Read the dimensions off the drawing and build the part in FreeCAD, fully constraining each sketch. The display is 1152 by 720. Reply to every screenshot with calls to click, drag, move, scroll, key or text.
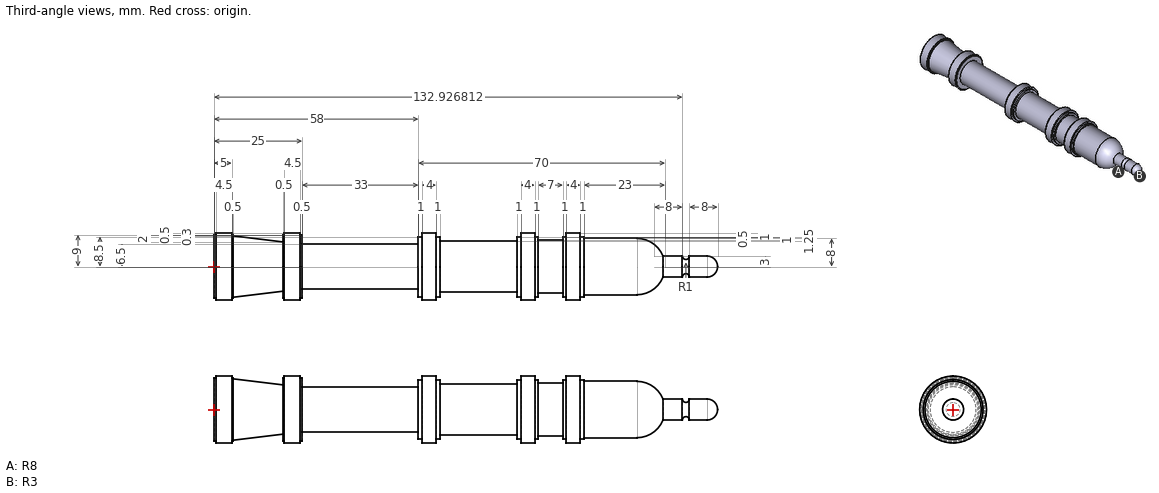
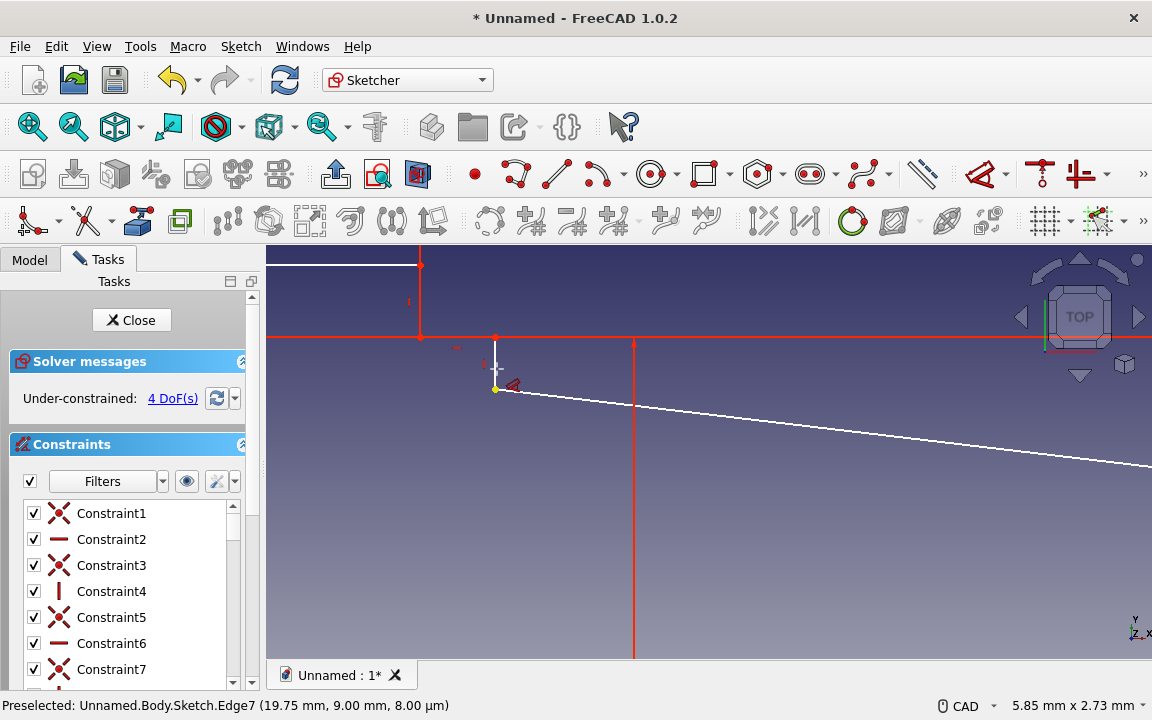
click(495, 369)
click(461, 363)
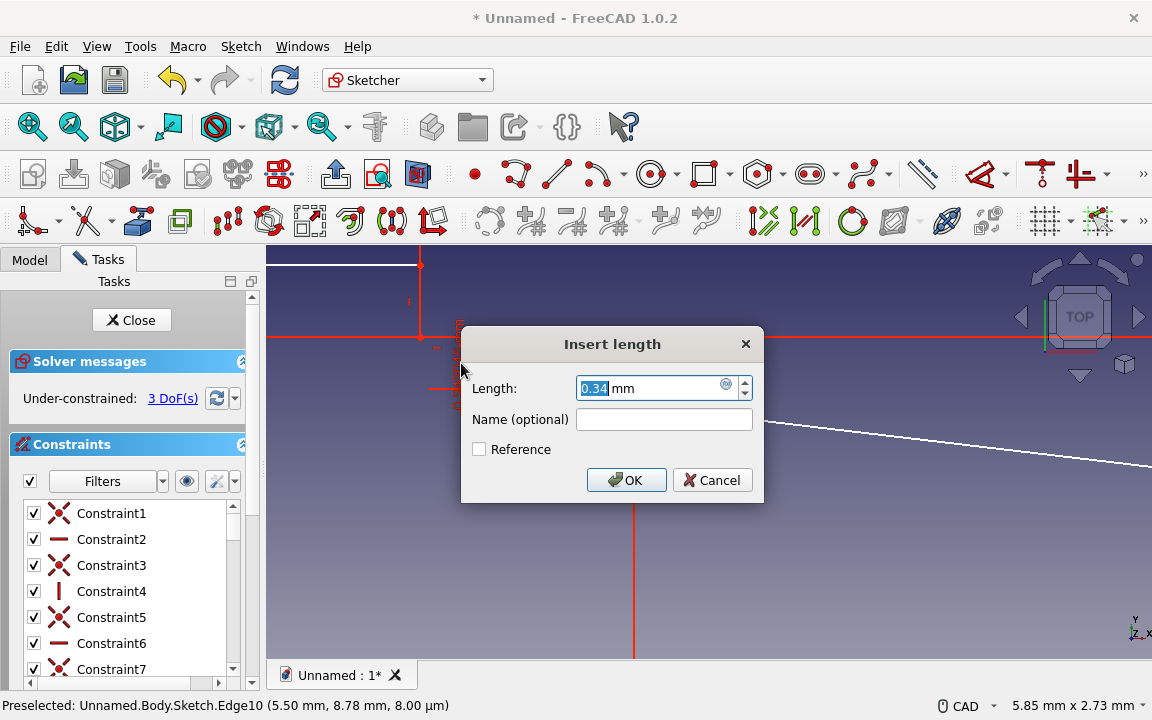
text(0.3)
key(Return)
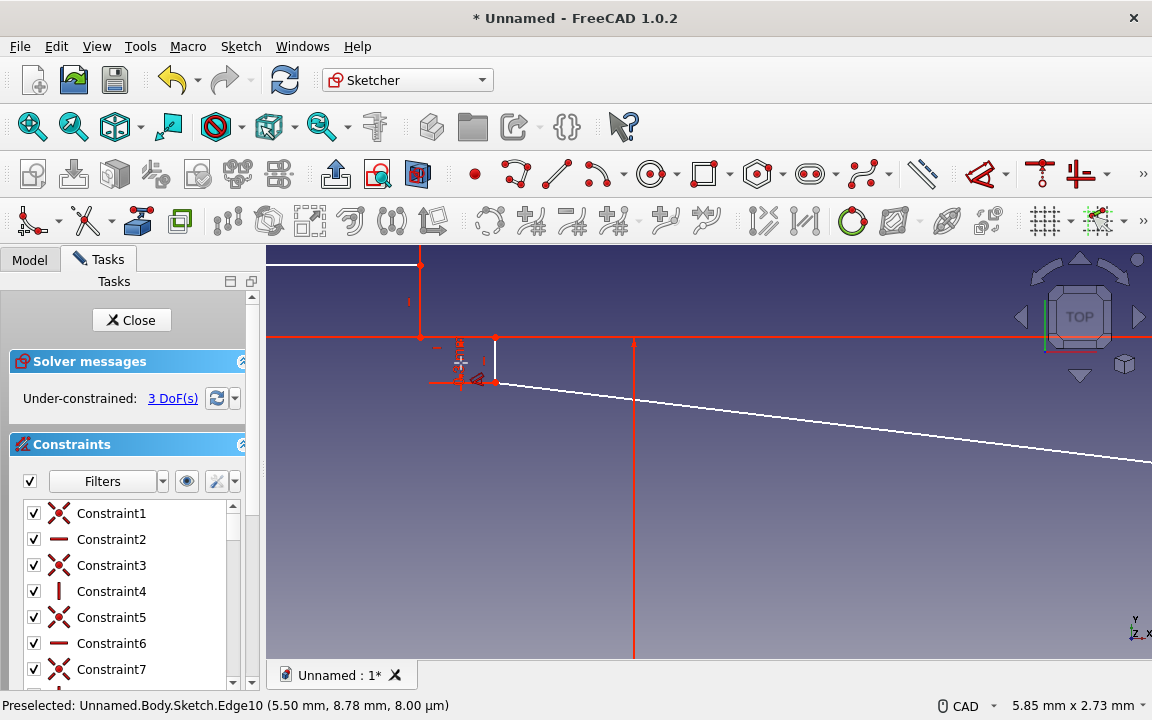
click(473, 337)
click(458, 303)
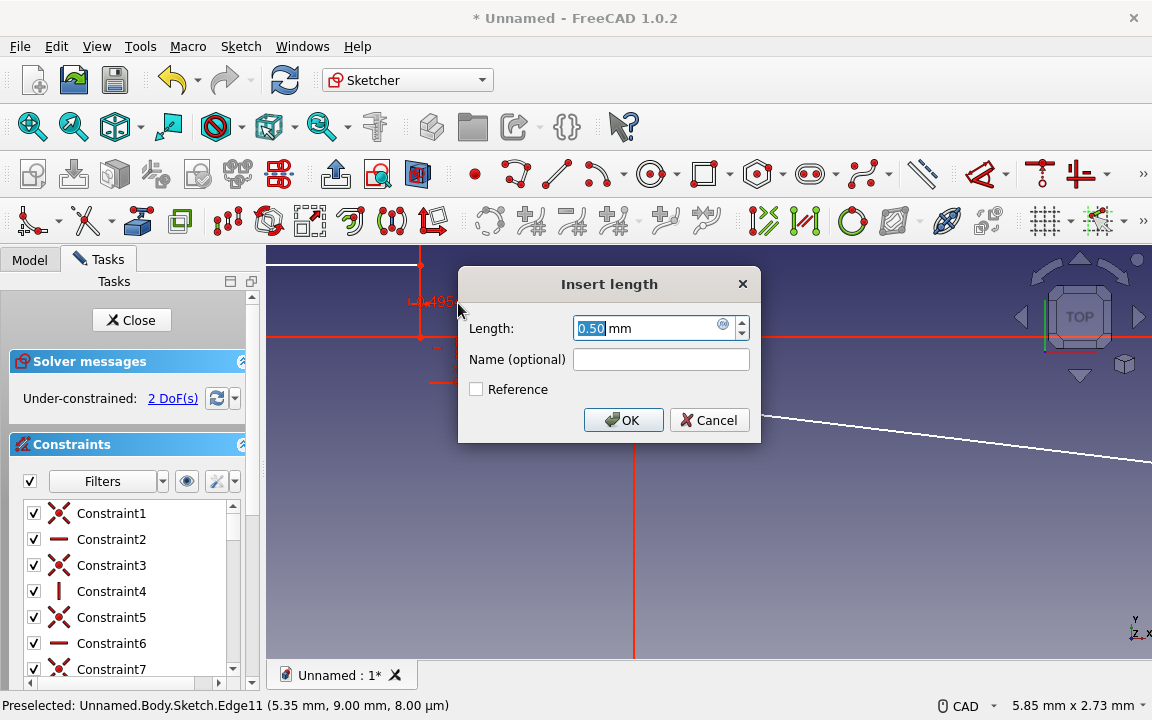
text(0.5)
key(Return)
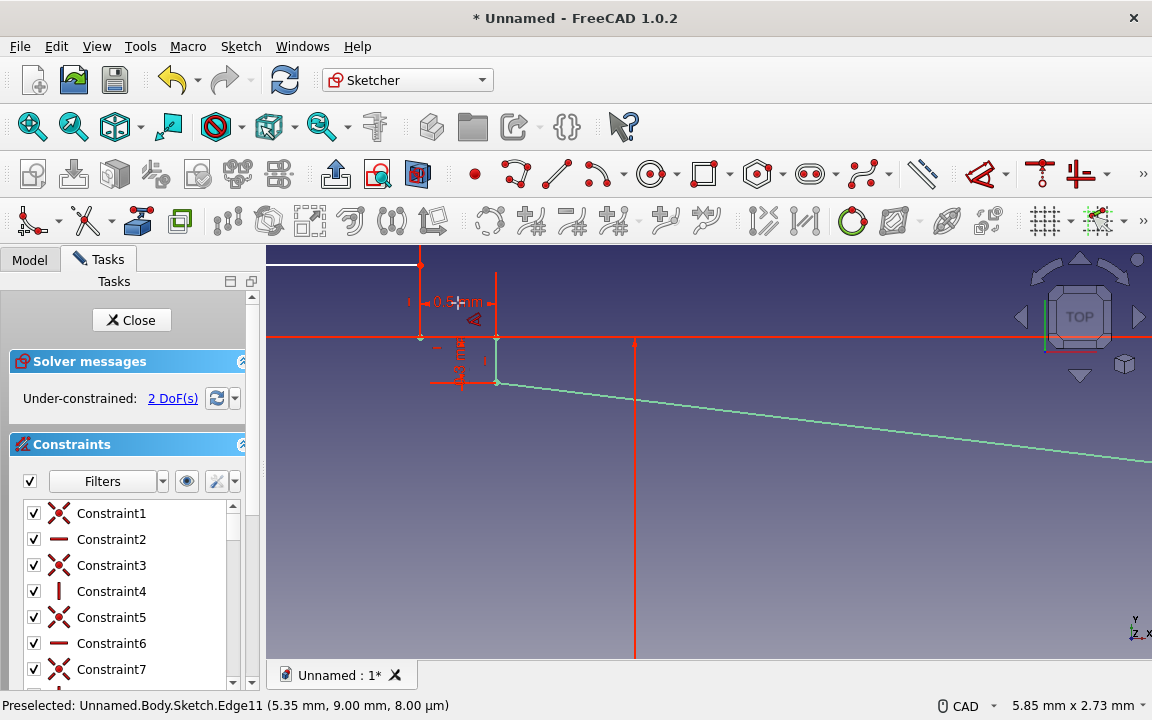
click(420, 316)
click(386, 305)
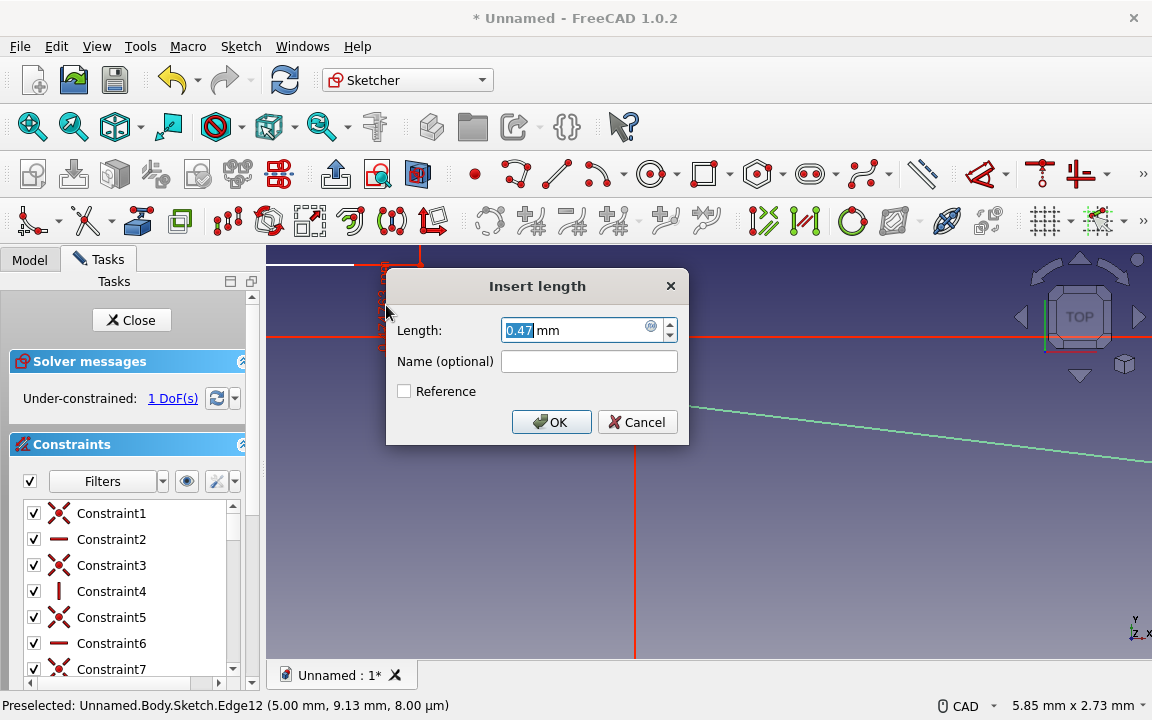
text(0.5)
key(Return)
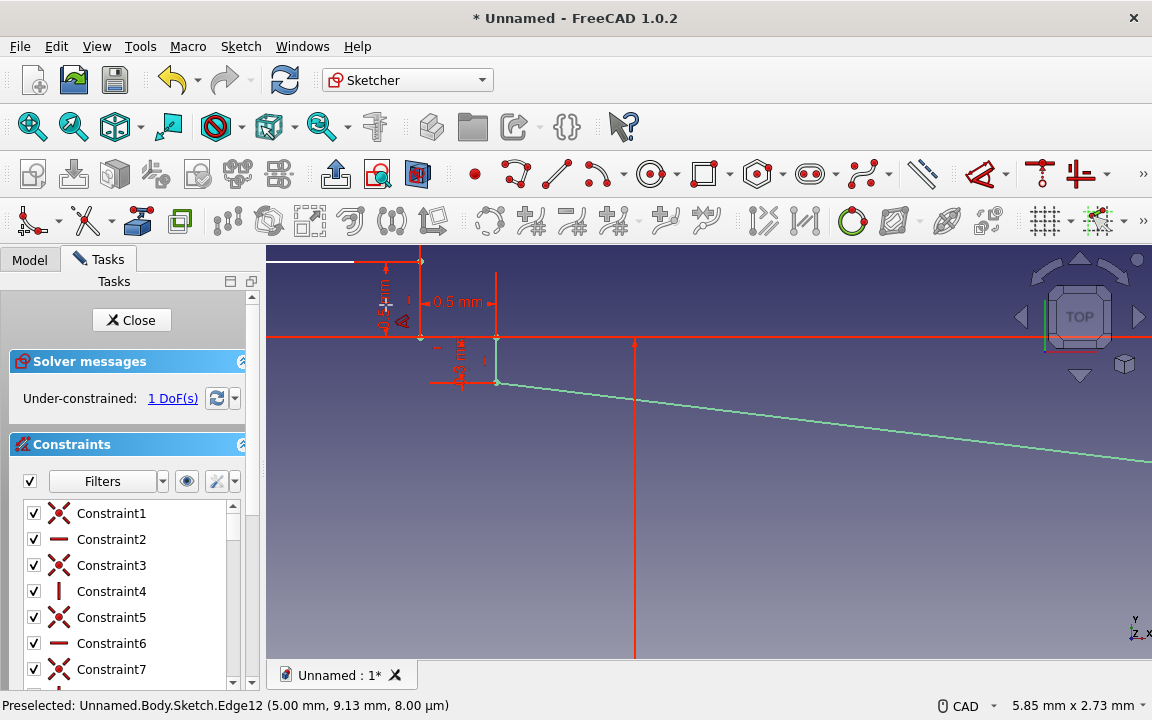
scroll(497, 369, down, 10)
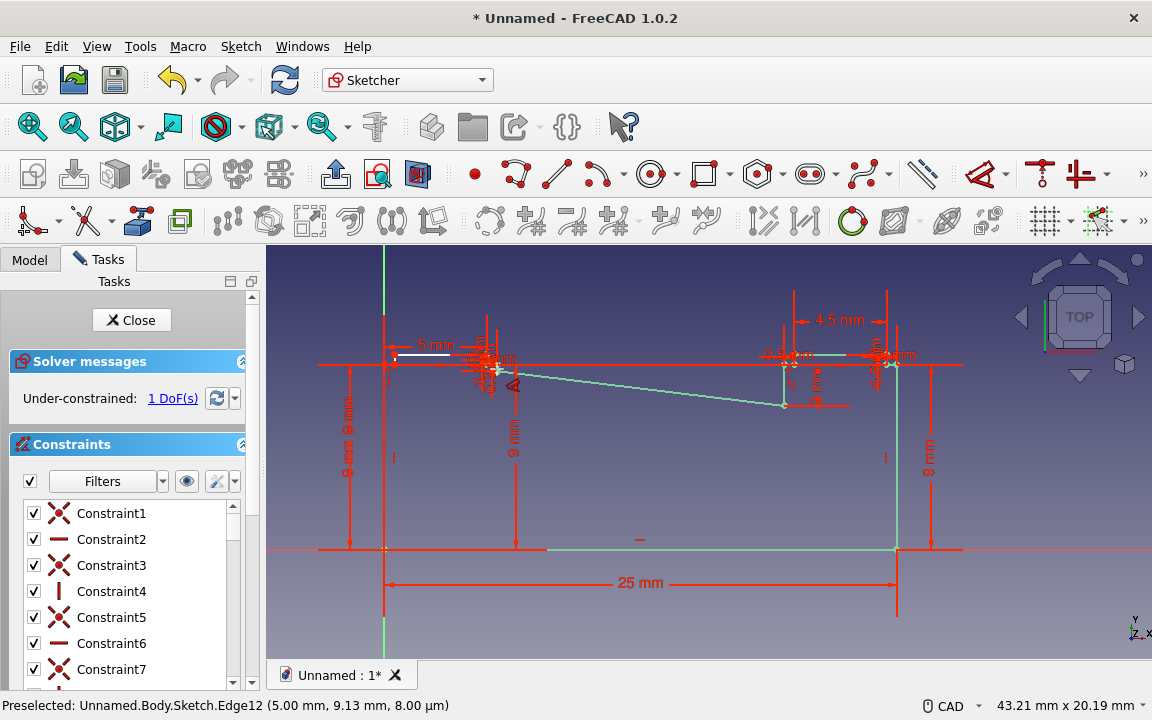
click(459, 355)
click(441, 321)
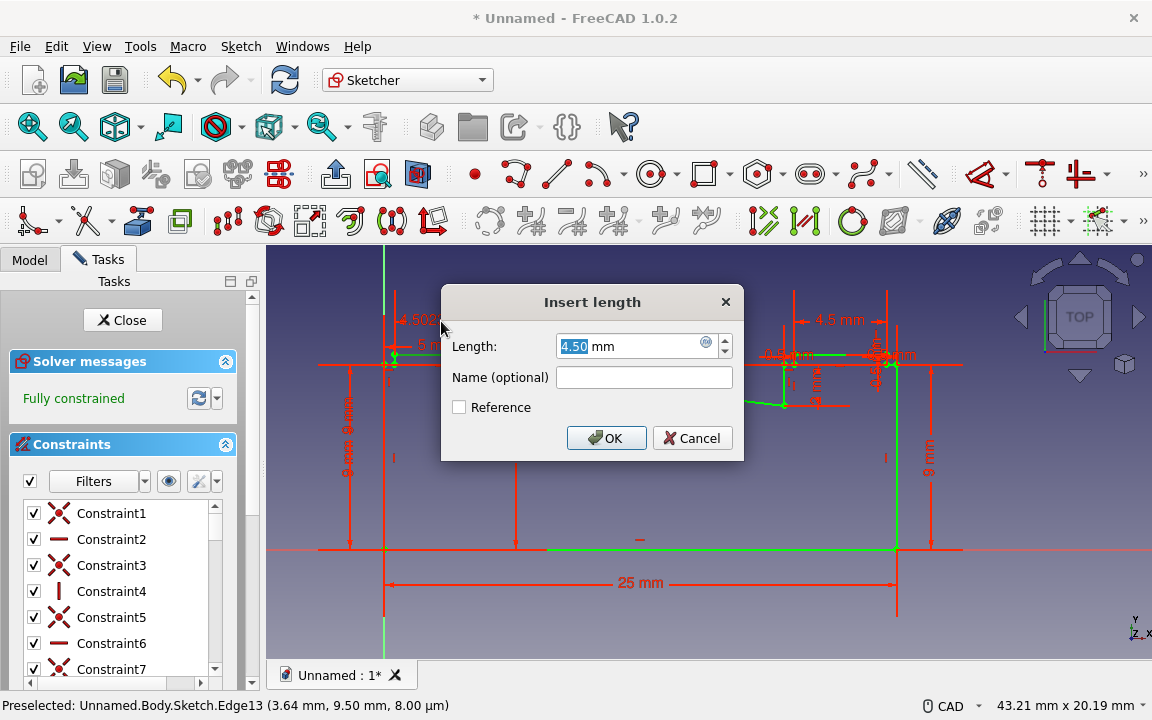
text(4.5)
key(Return)
key(Escape)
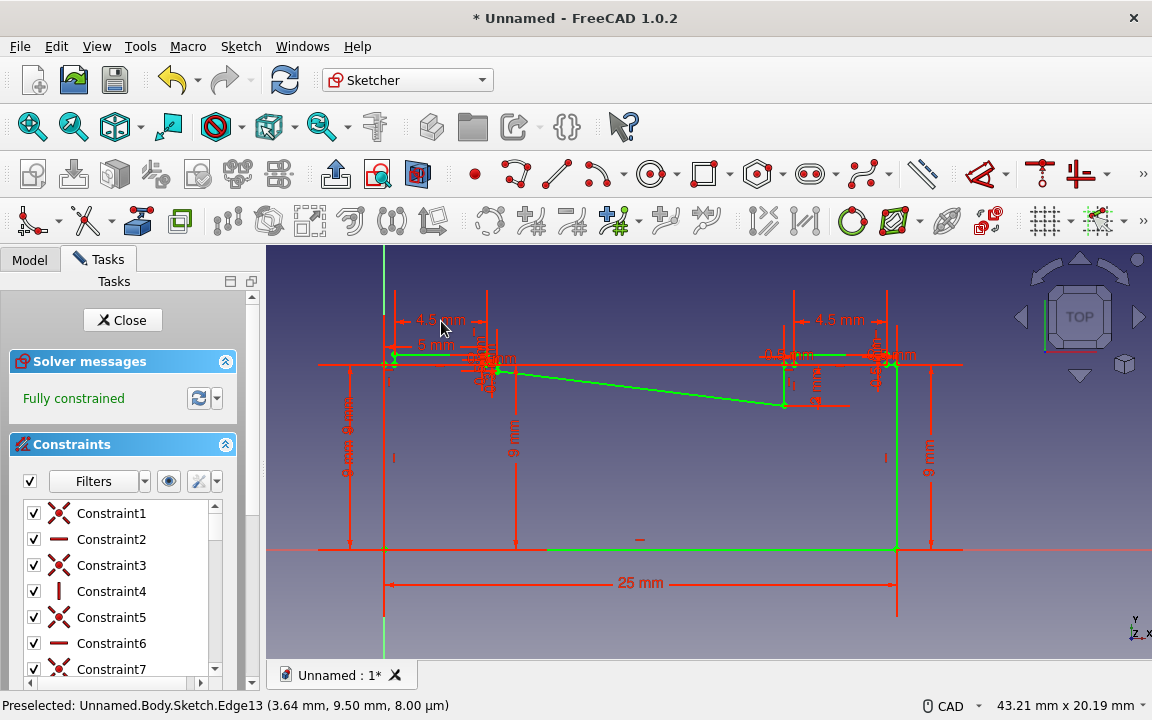
click(123, 320)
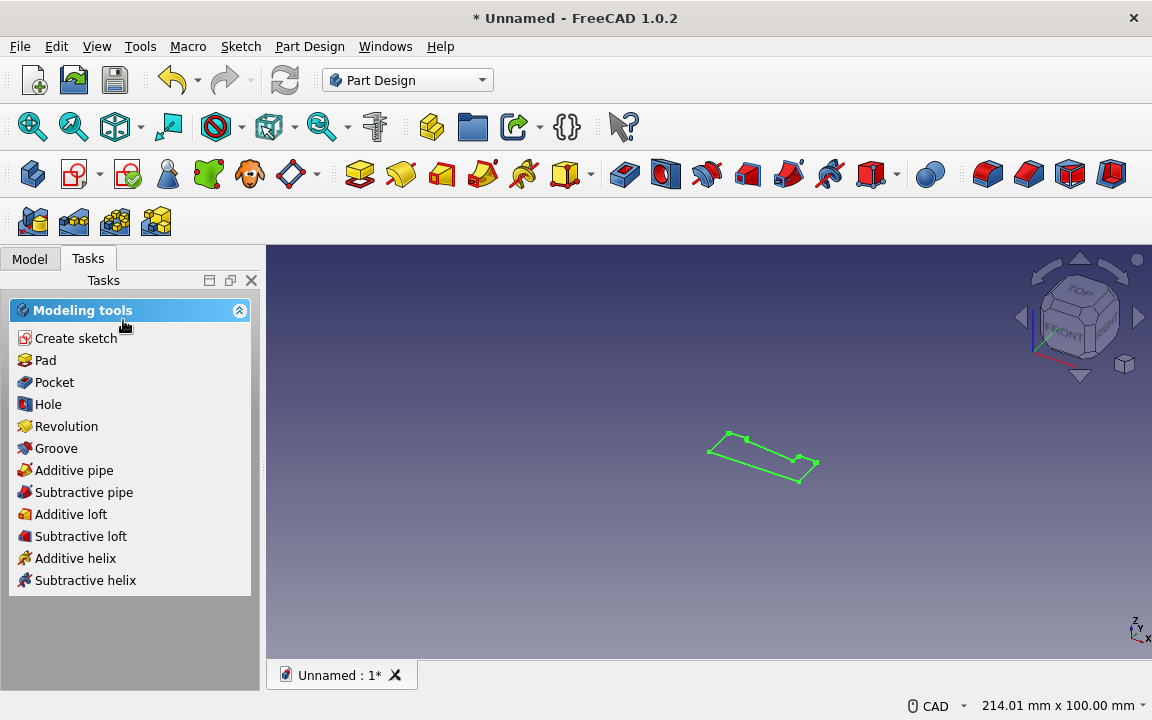
click(401, 174)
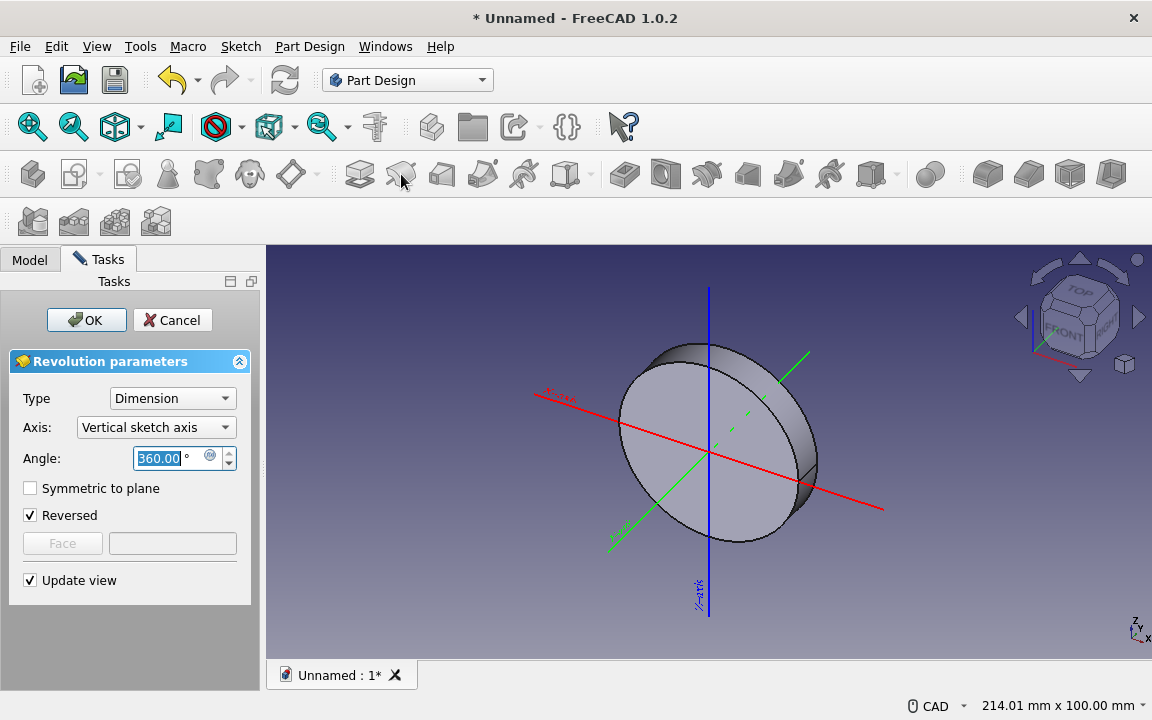
click(157, 428)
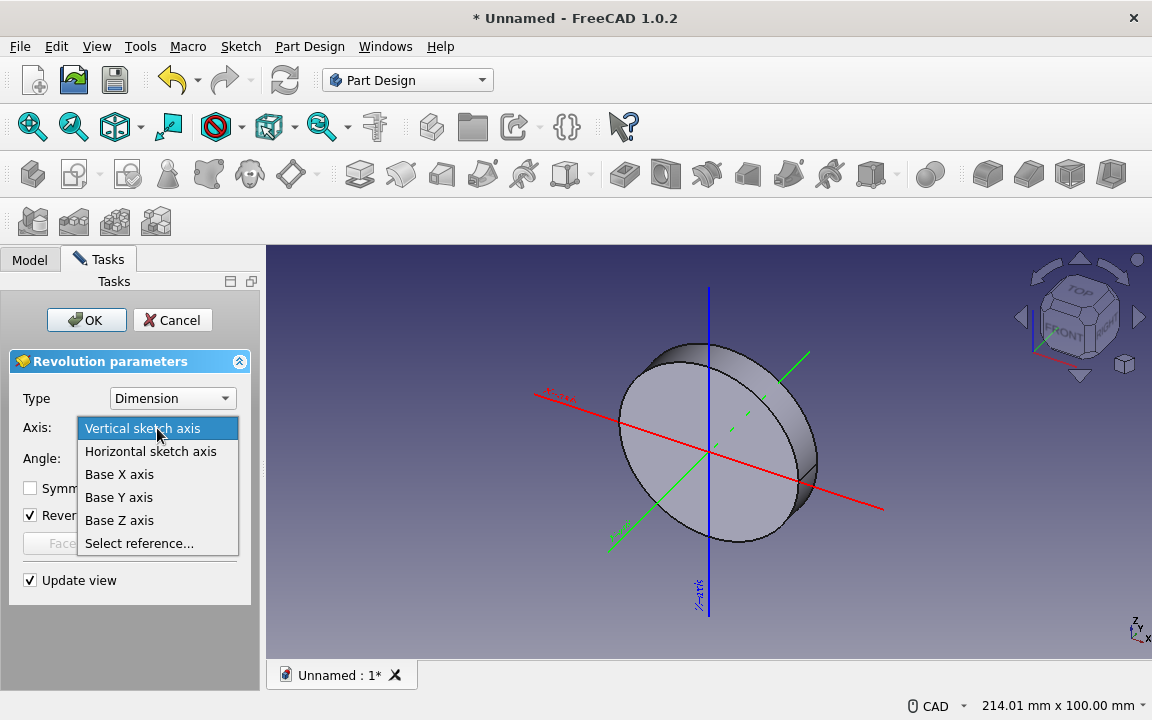
click(156, 452)